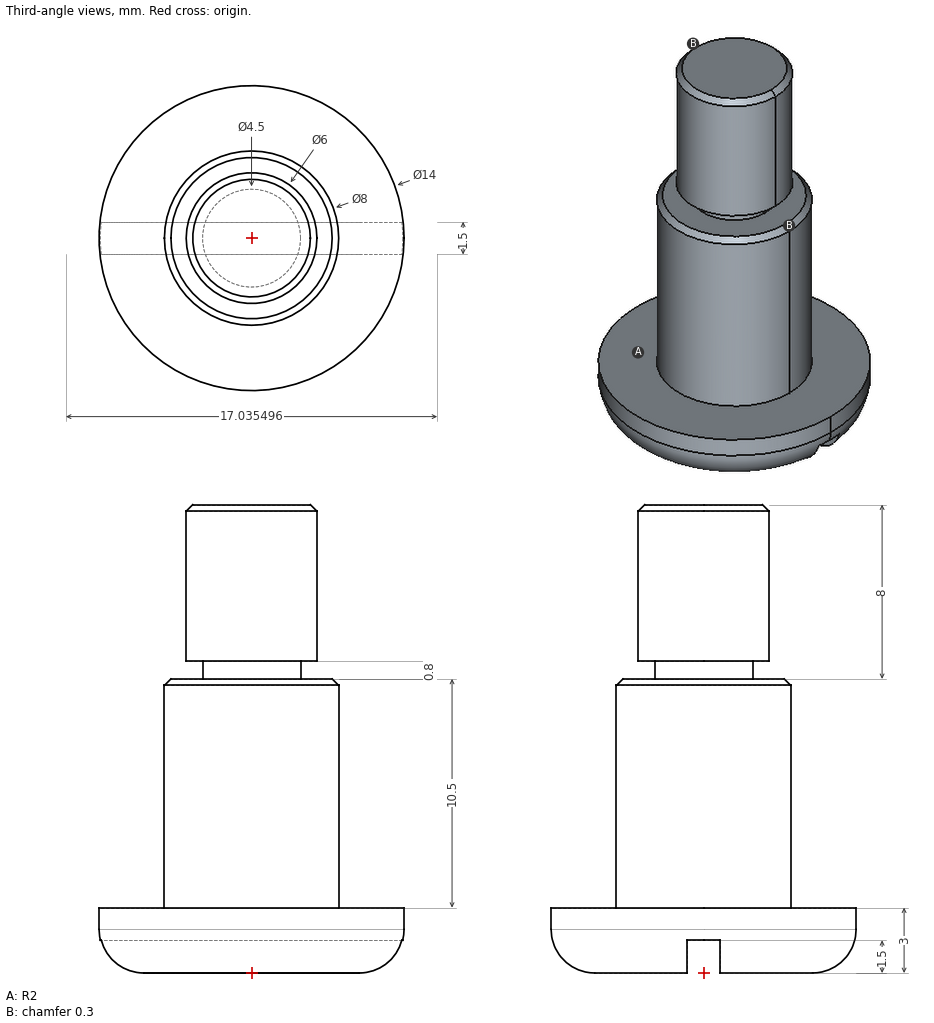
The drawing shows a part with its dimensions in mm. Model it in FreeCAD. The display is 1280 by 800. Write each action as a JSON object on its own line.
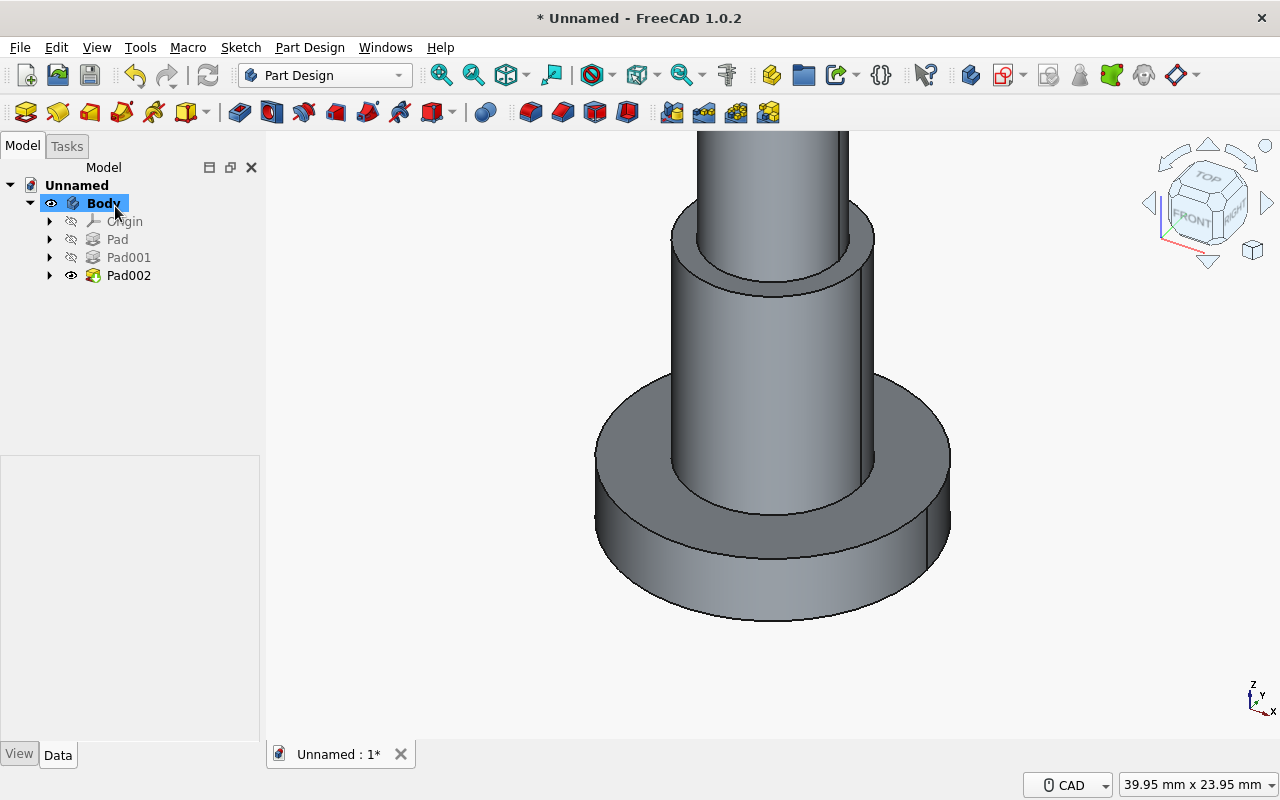
{"action": "left_click", "coordinate": [442, 76]}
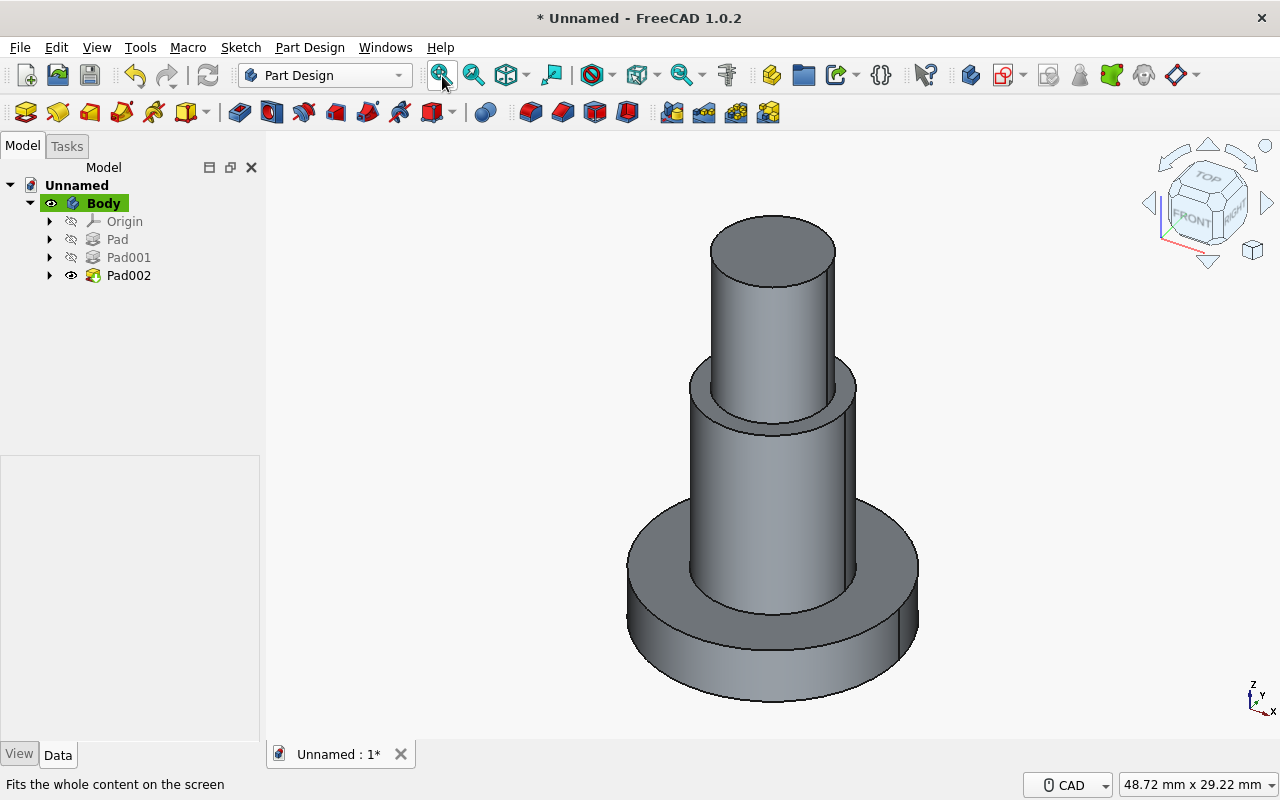
{"action": "left_click", "coordinate": [699, 378]}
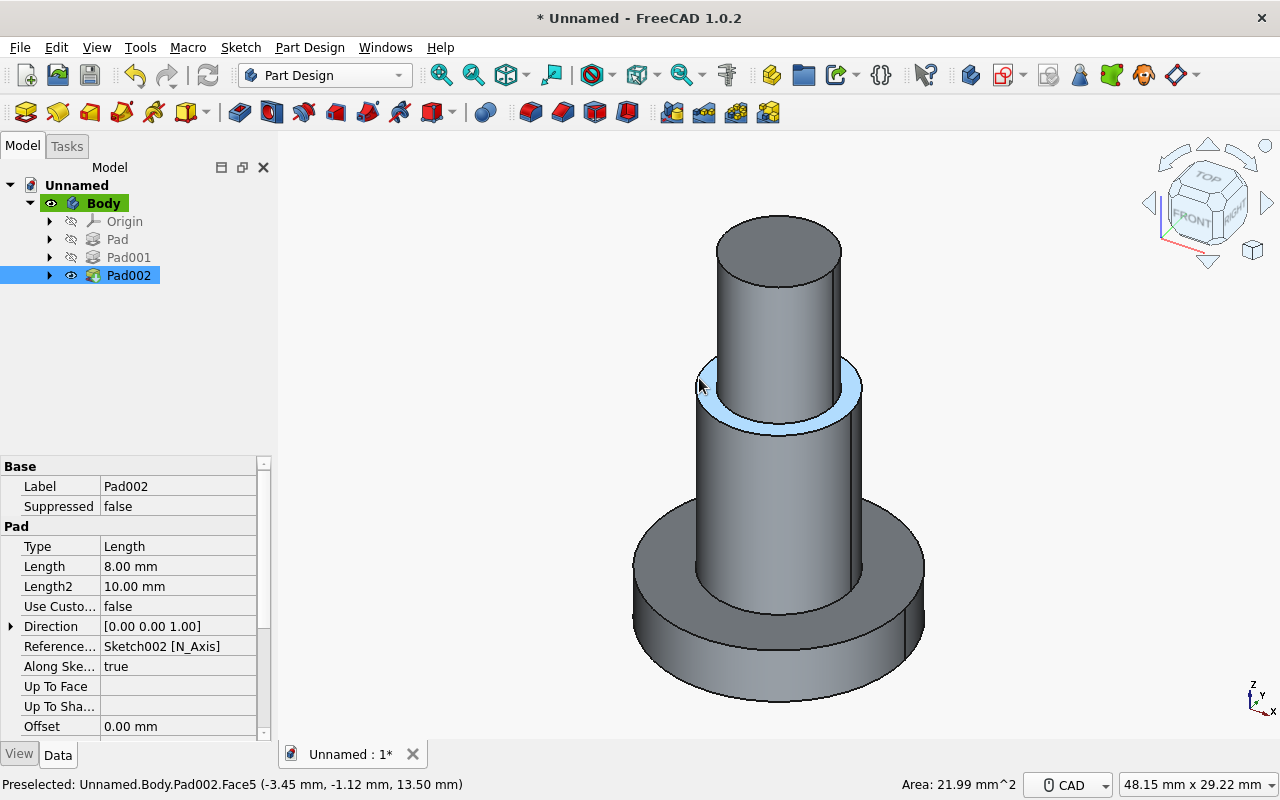
{"action": "left_click", "coordinate": [1004, 76]}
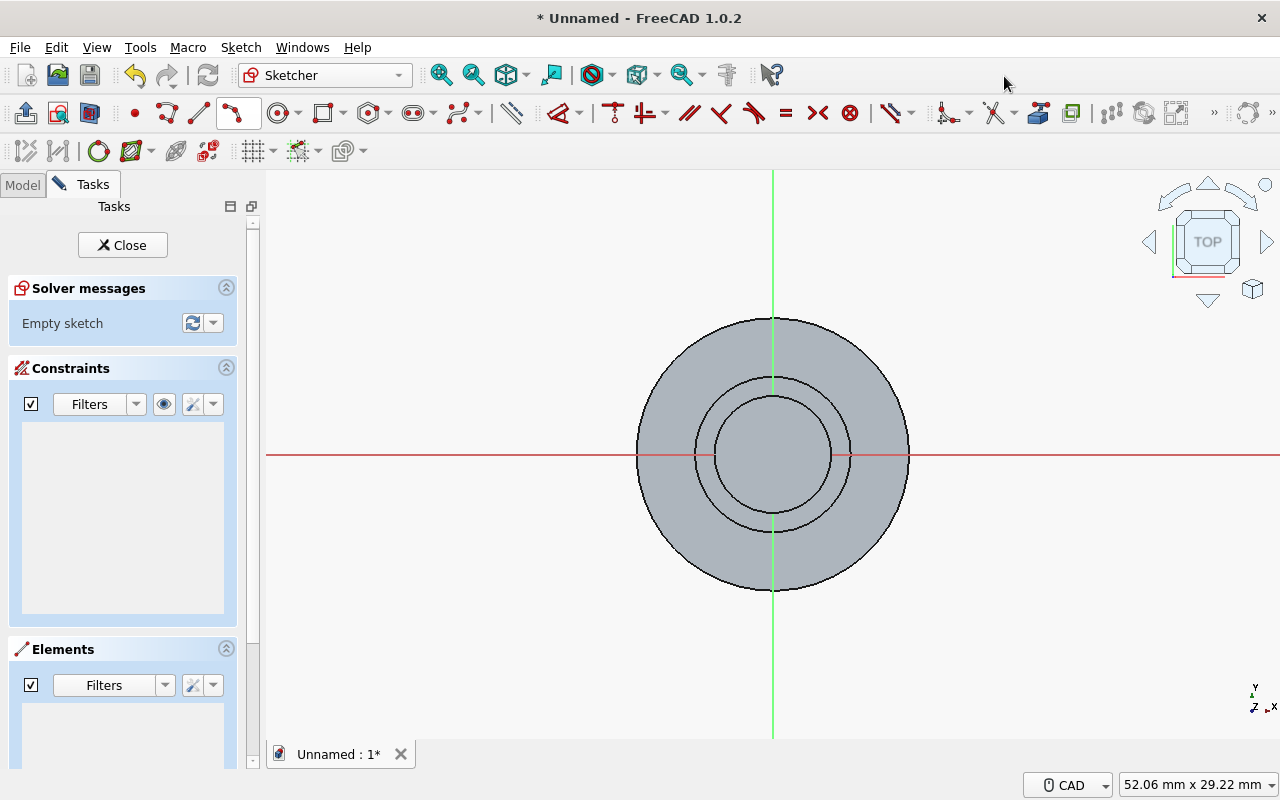
{"action": "scroll", "coordinate": [802, 455], "scroll_direction": "up", "scroll_amount": 6}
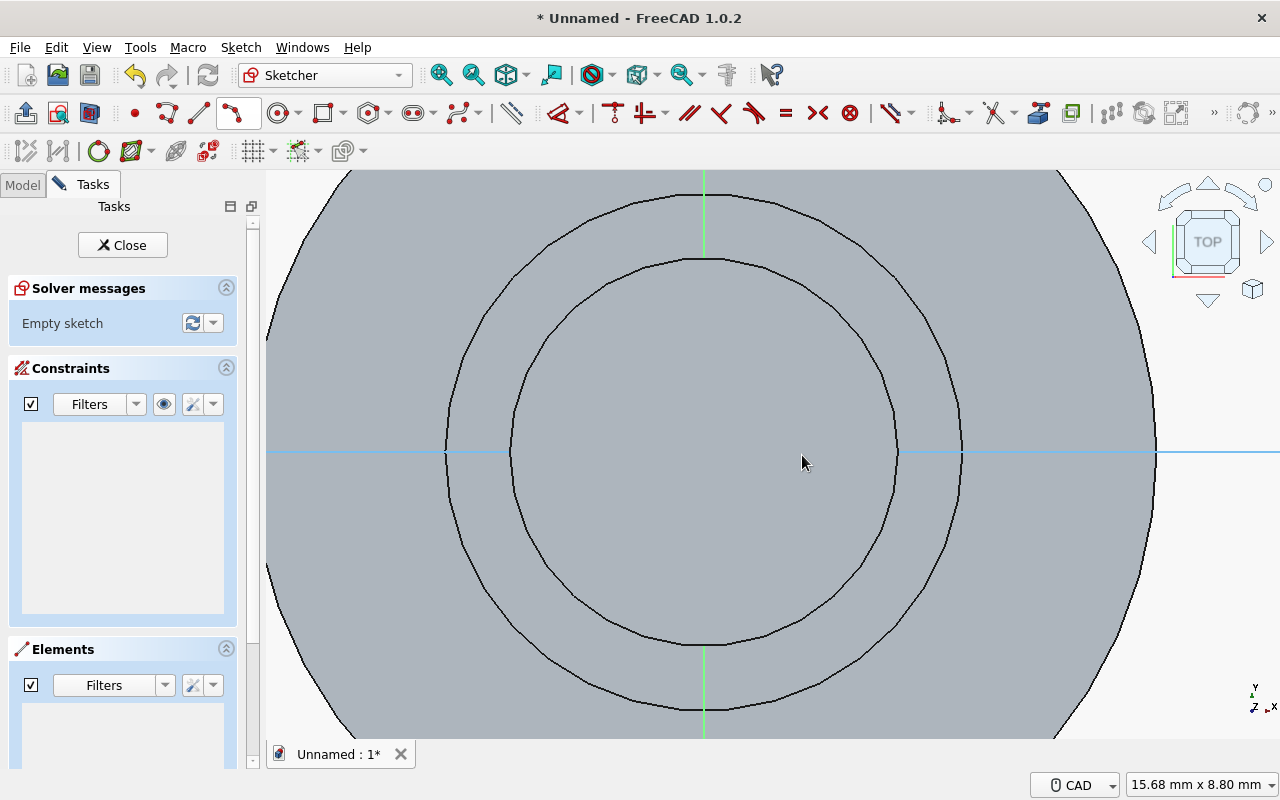
{"action": "left_click", "coordinate": [278, 114]}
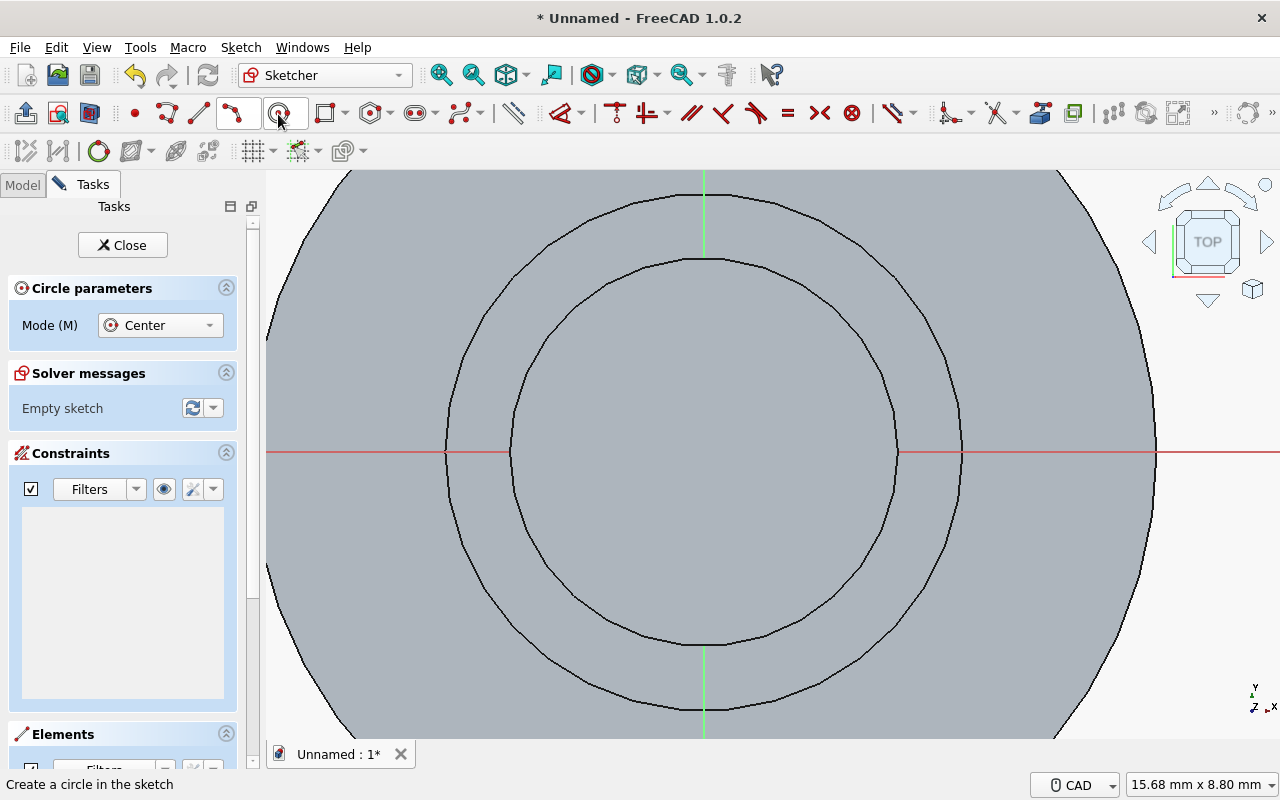
{"action": "left_click", "coordinate": [704, 452]}
{"action": "left_click", "coordinate": [841, 315]}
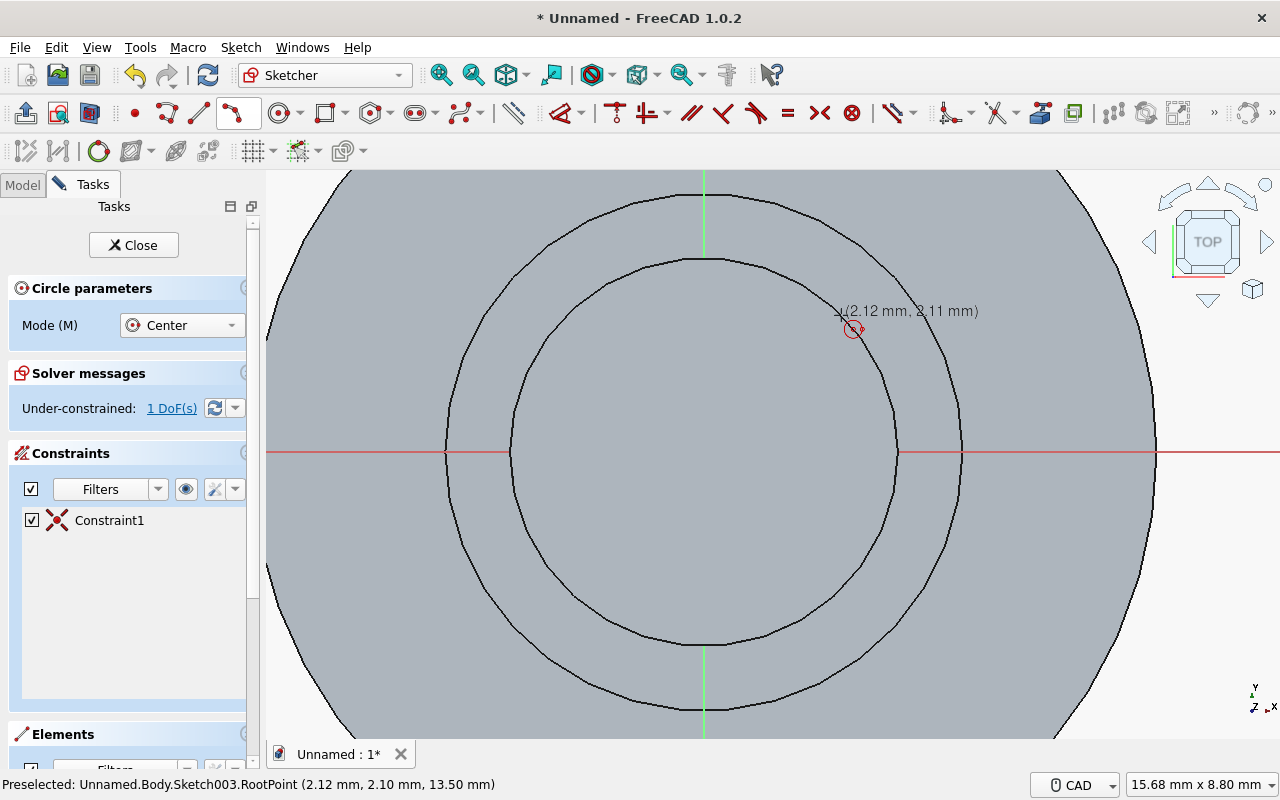
{"action": "left_click", "coordinate": [704, 452]}
{"action": "left_click", "coordinate": [807, 349]}
{"action": "key", "text": "Escape"}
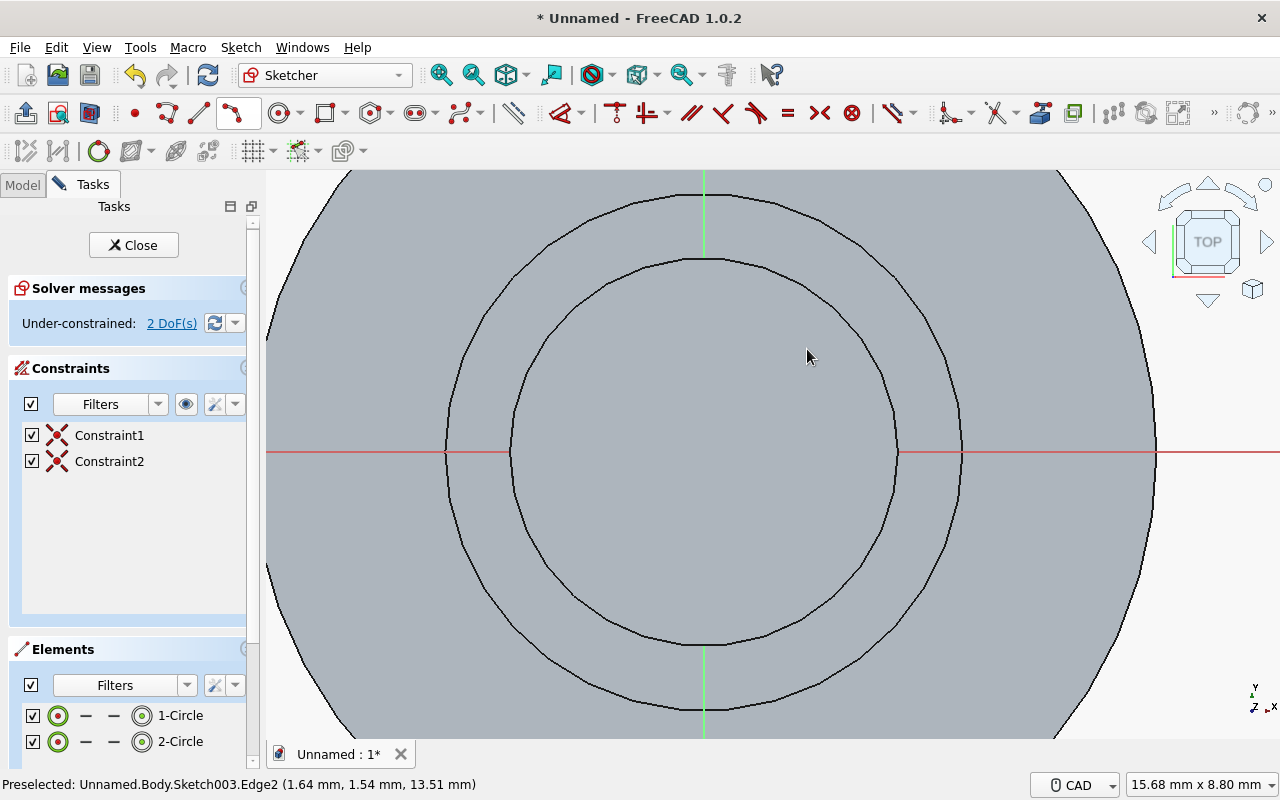
{"action": "left_click", "coordinate": [560, 114]}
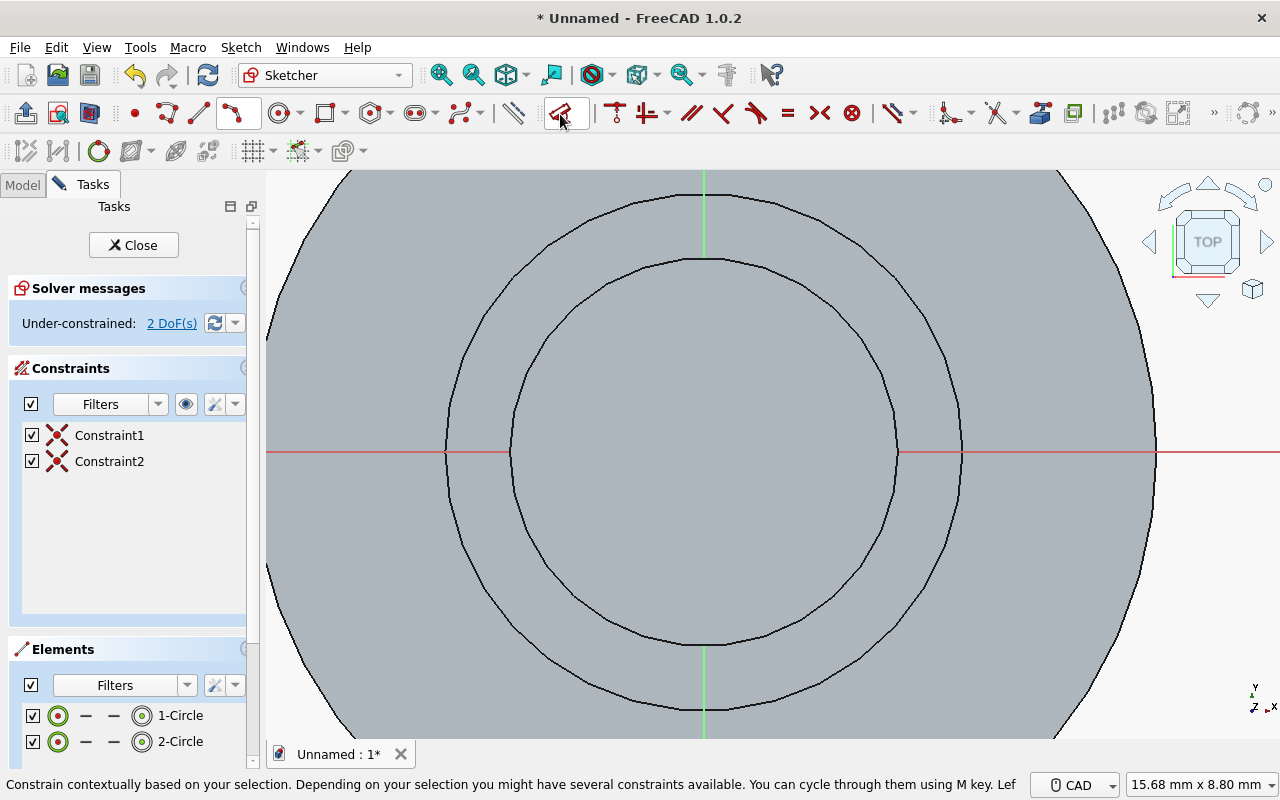
{"action": "left_click", "coordinate": [840, 315]}
{"action": "left_click", "coordinate": [863, 292]}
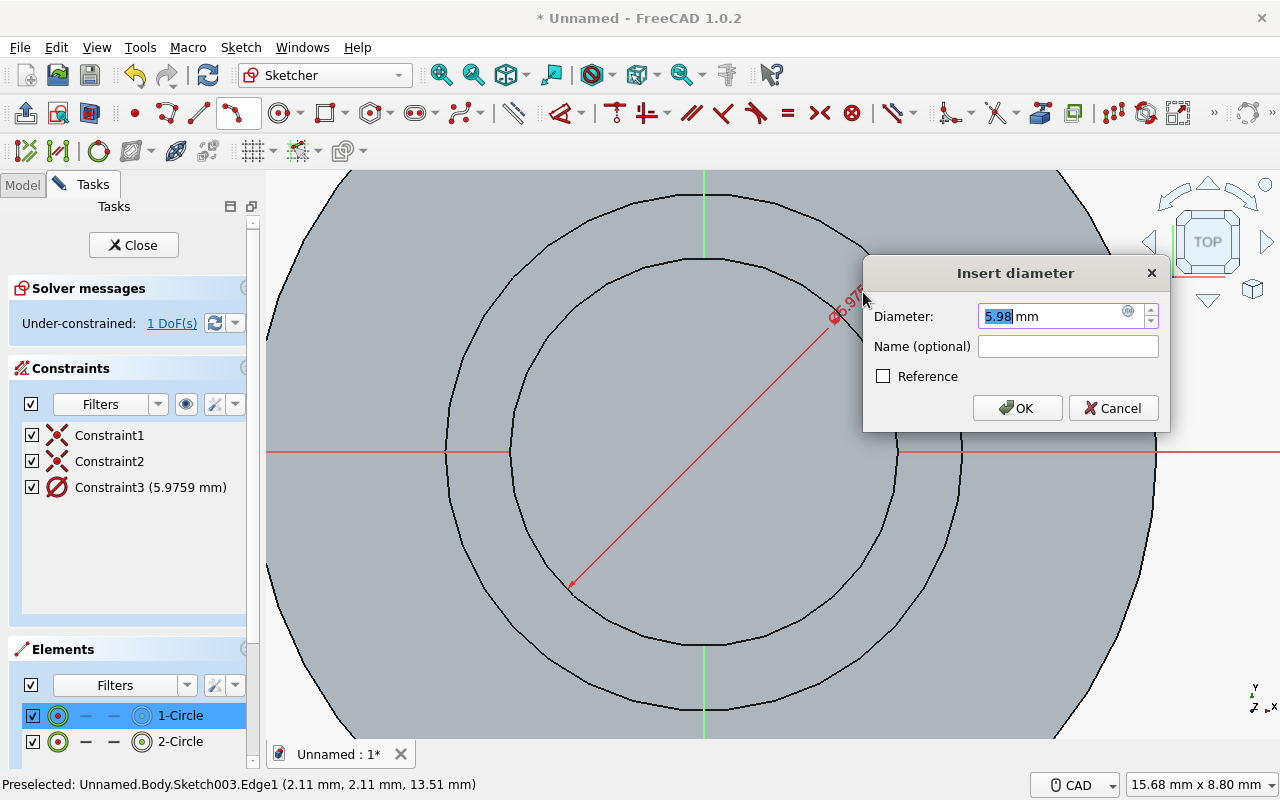
{"action": "type", "text": "6"}
{"action": "key", "text": "Return"}